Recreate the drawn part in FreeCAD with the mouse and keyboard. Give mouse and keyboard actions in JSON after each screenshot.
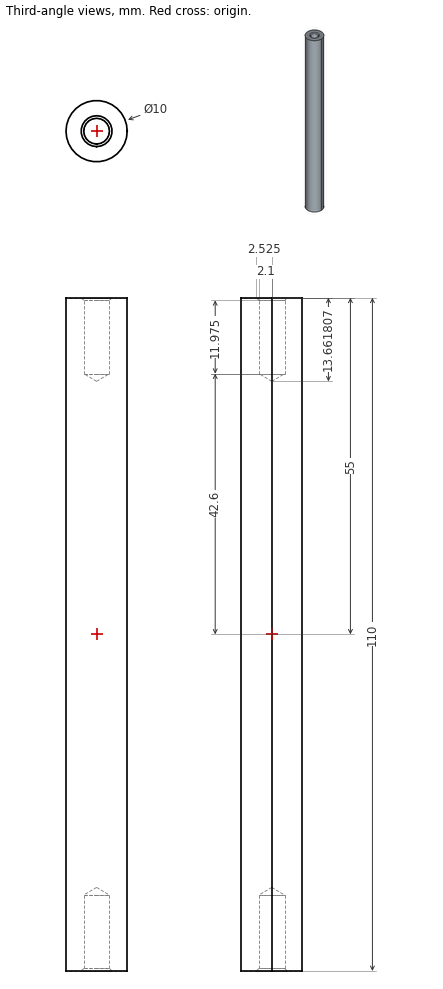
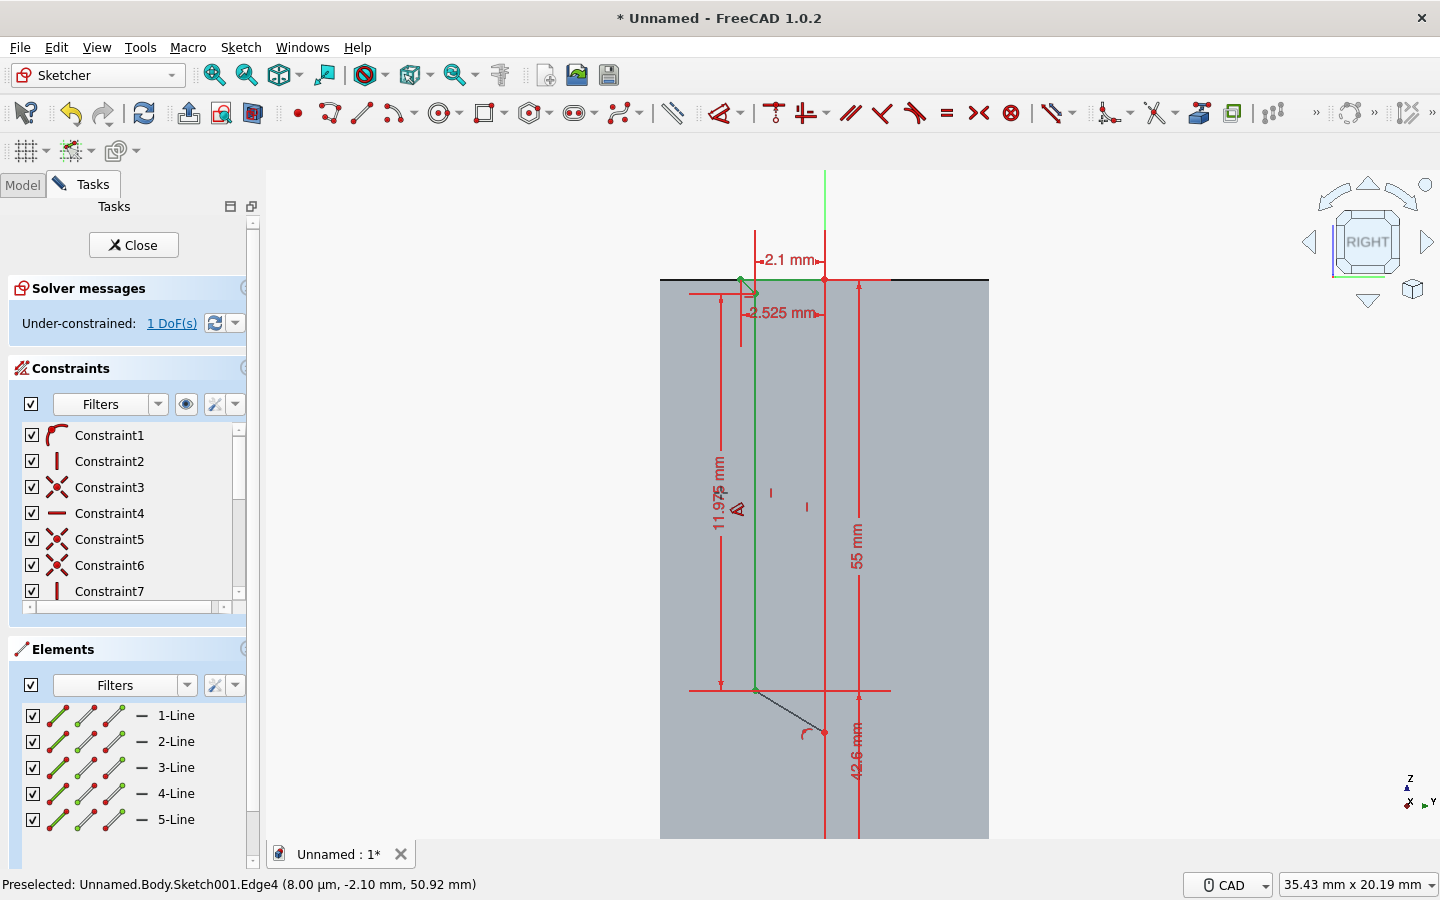
{"action": "left_click", "coordinate": [825, 597]}
{"action": "left_click", "coordinate": [859, 506]}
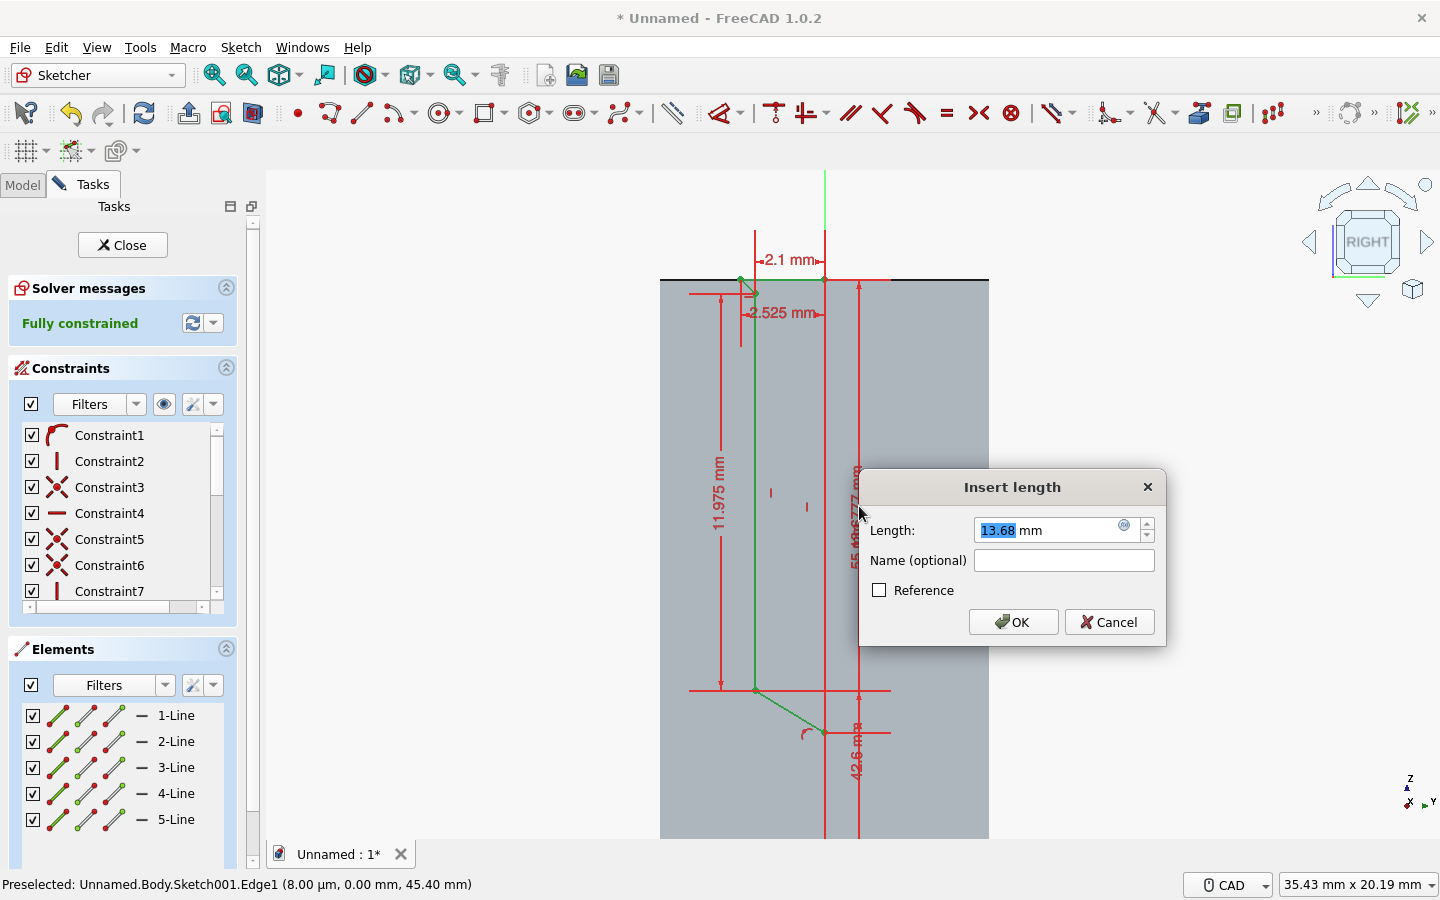
{"action": "type", "text": "13.661807"}
{"action": "key", "text": "Return"}
{"action": "key", "text": "Escape"}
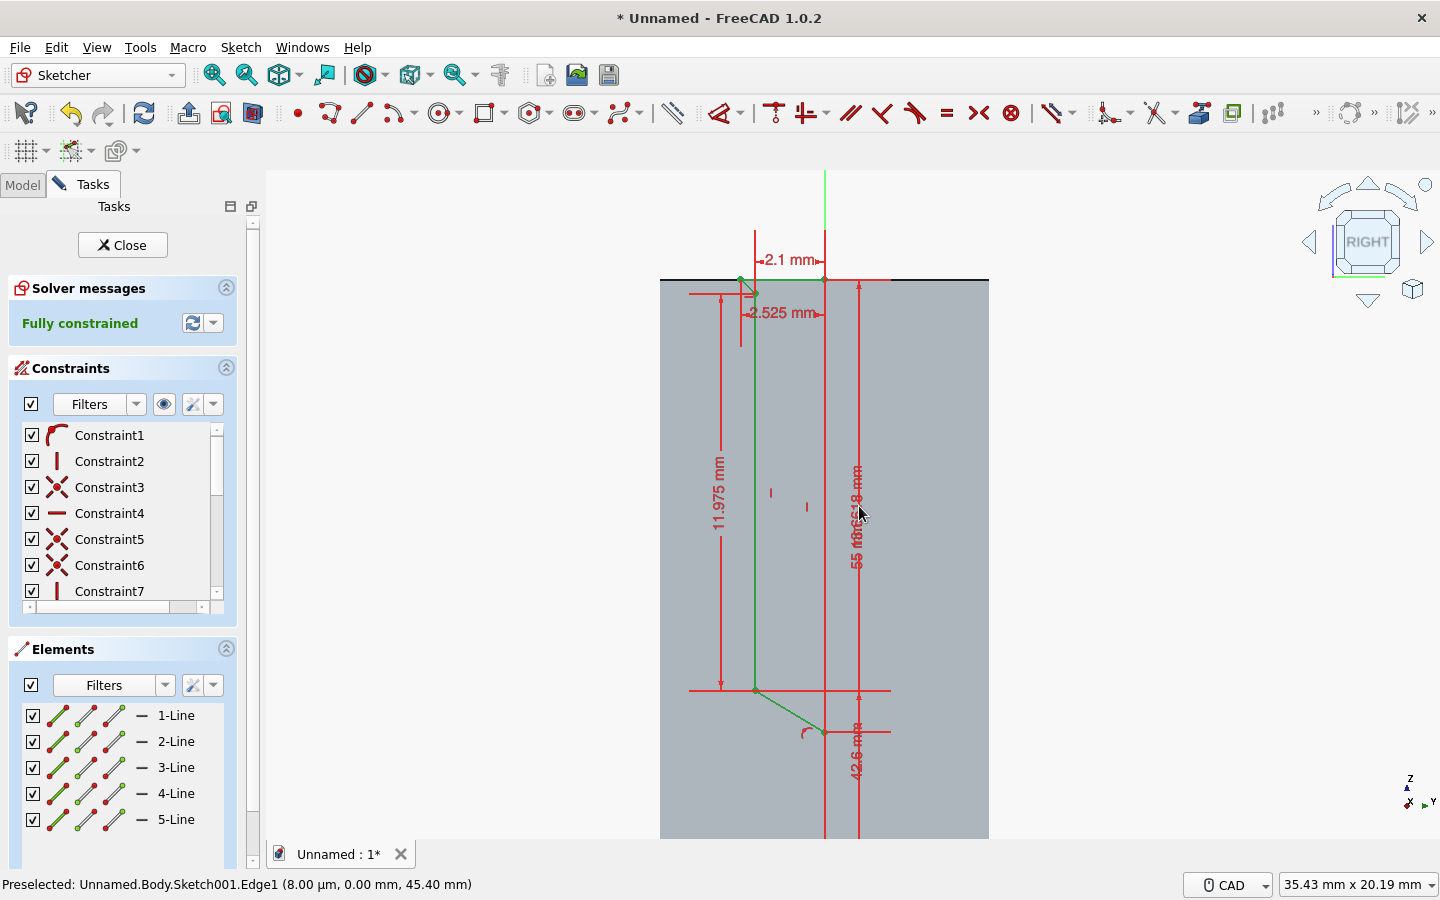
{"action": "left_click", "coordinate": [123, 245]}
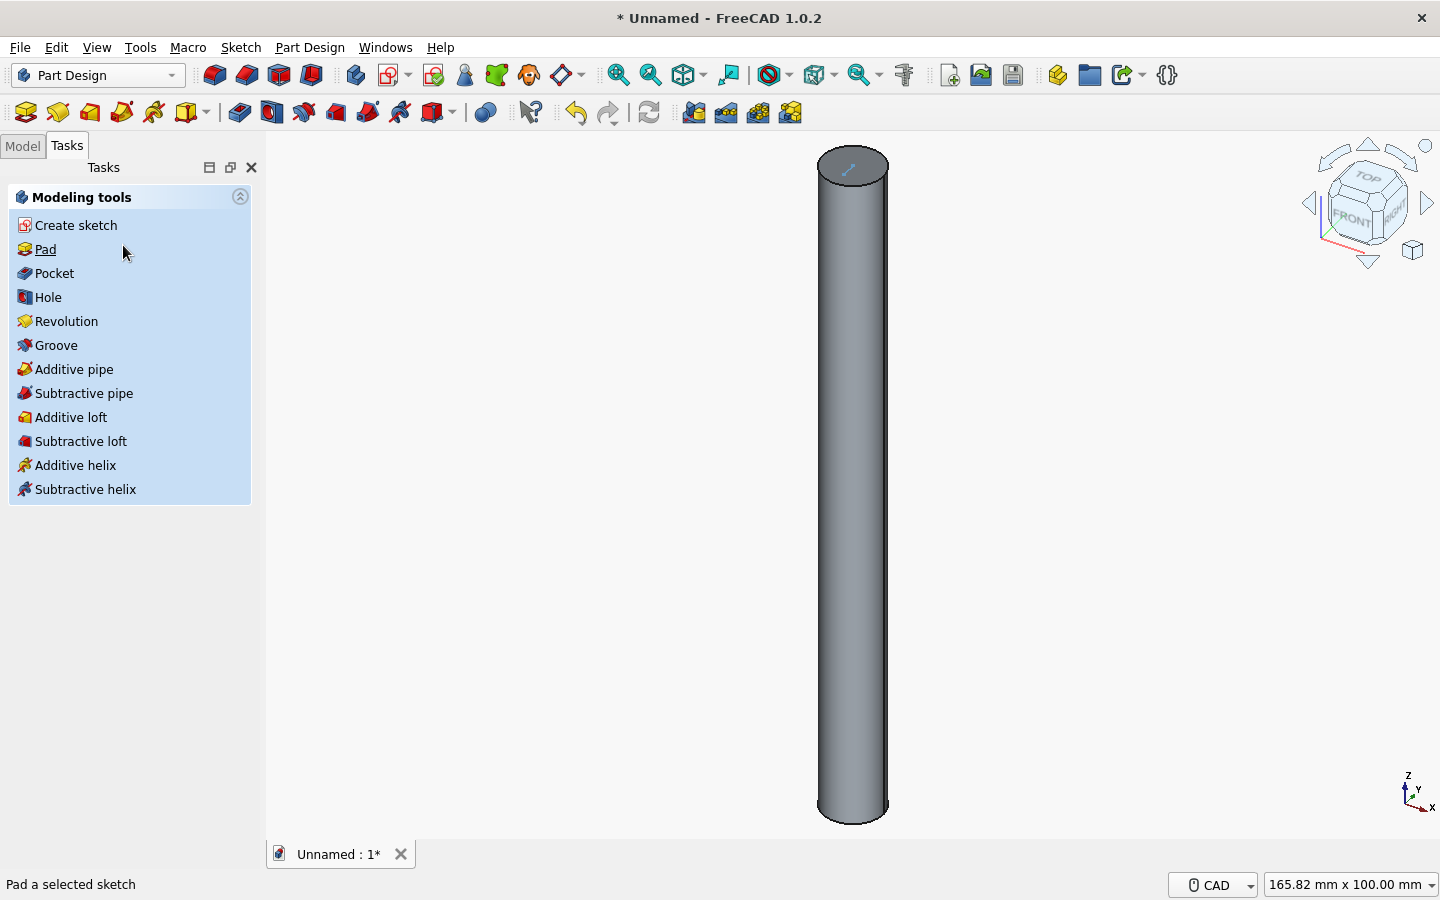
{"action": "left_click", "coordinate": [304, 112]}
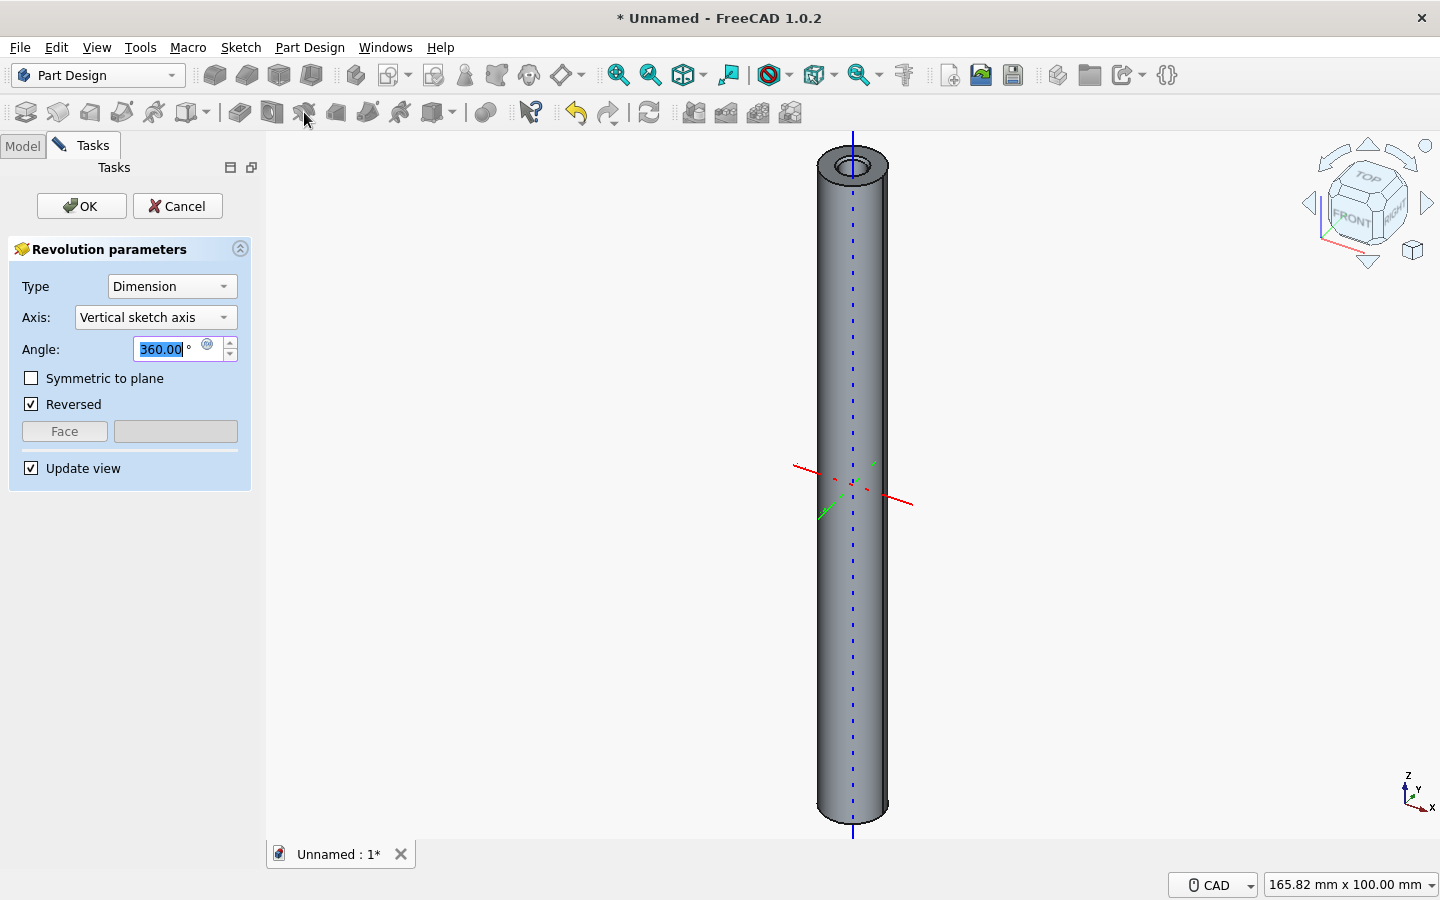
{"action": "left_click", "coordinate": [82, 206]}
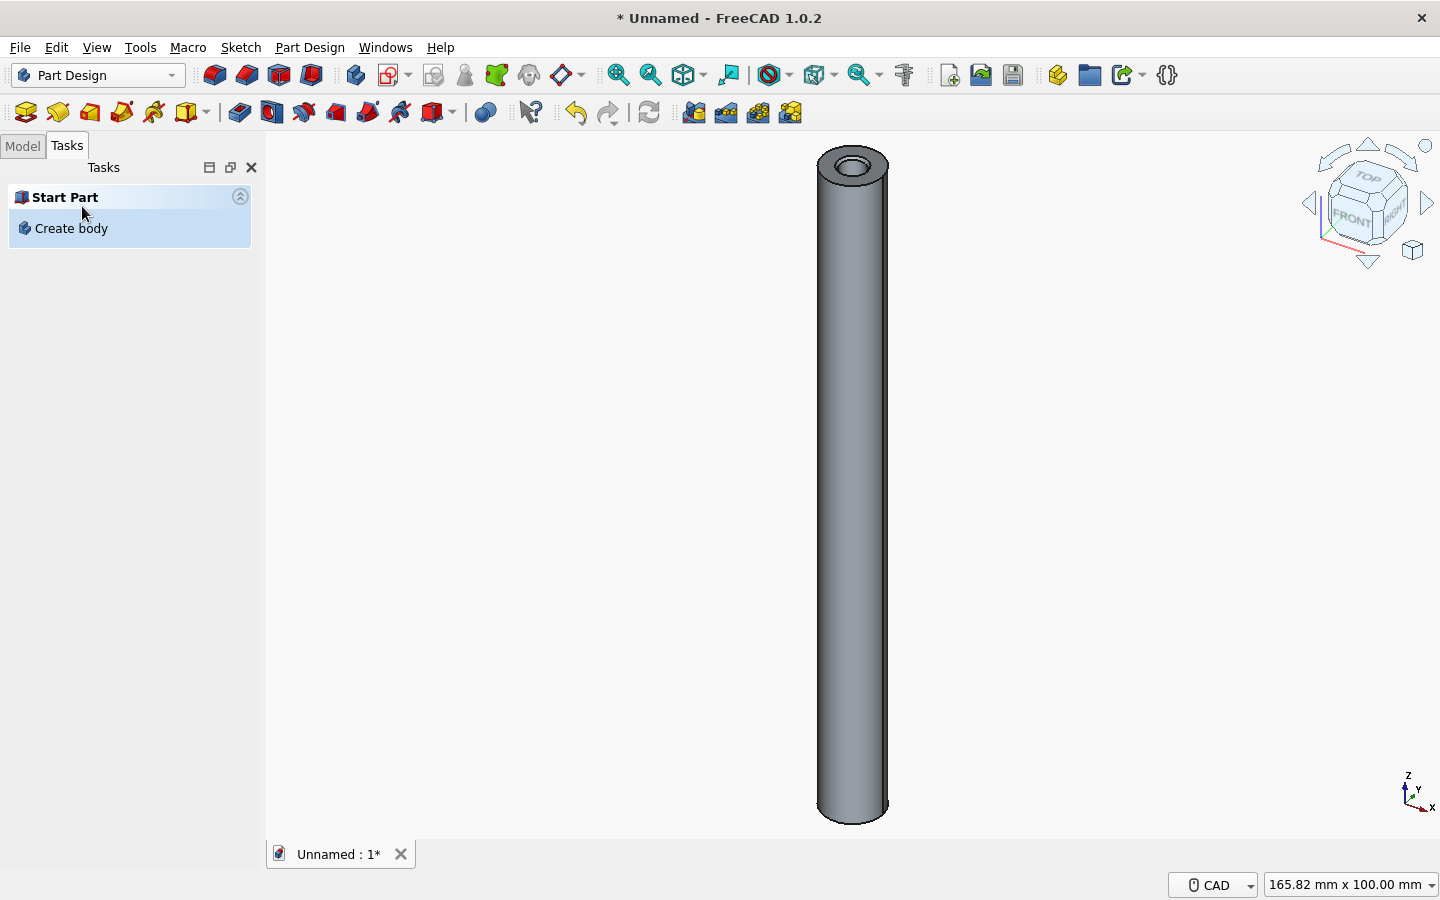
{"action": "left_click", "coordinate": [23, 145]}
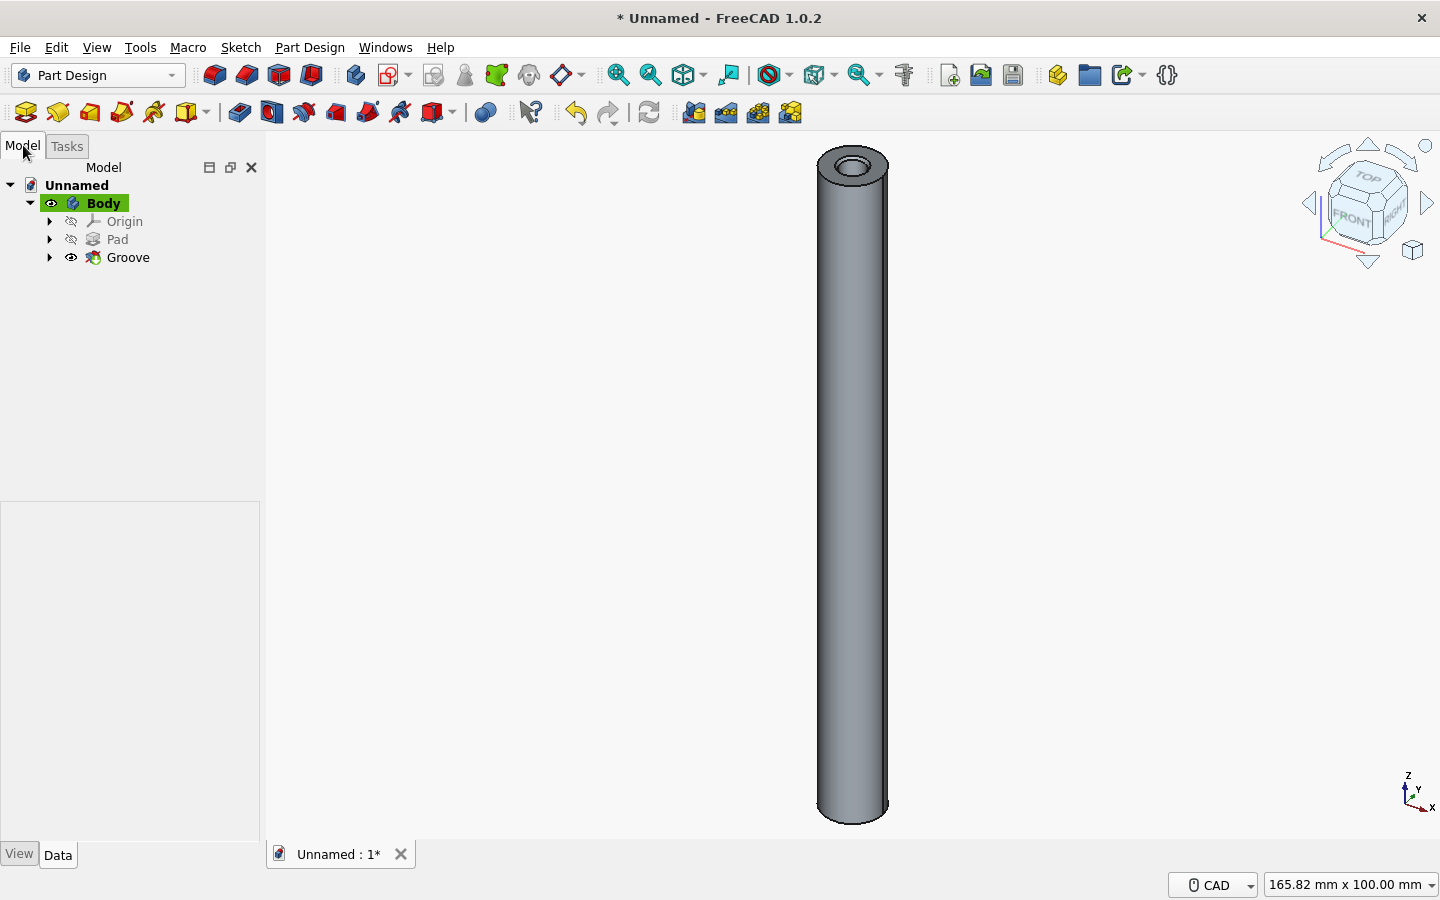
{"action": "left_click", "coordinate": [116, 257]}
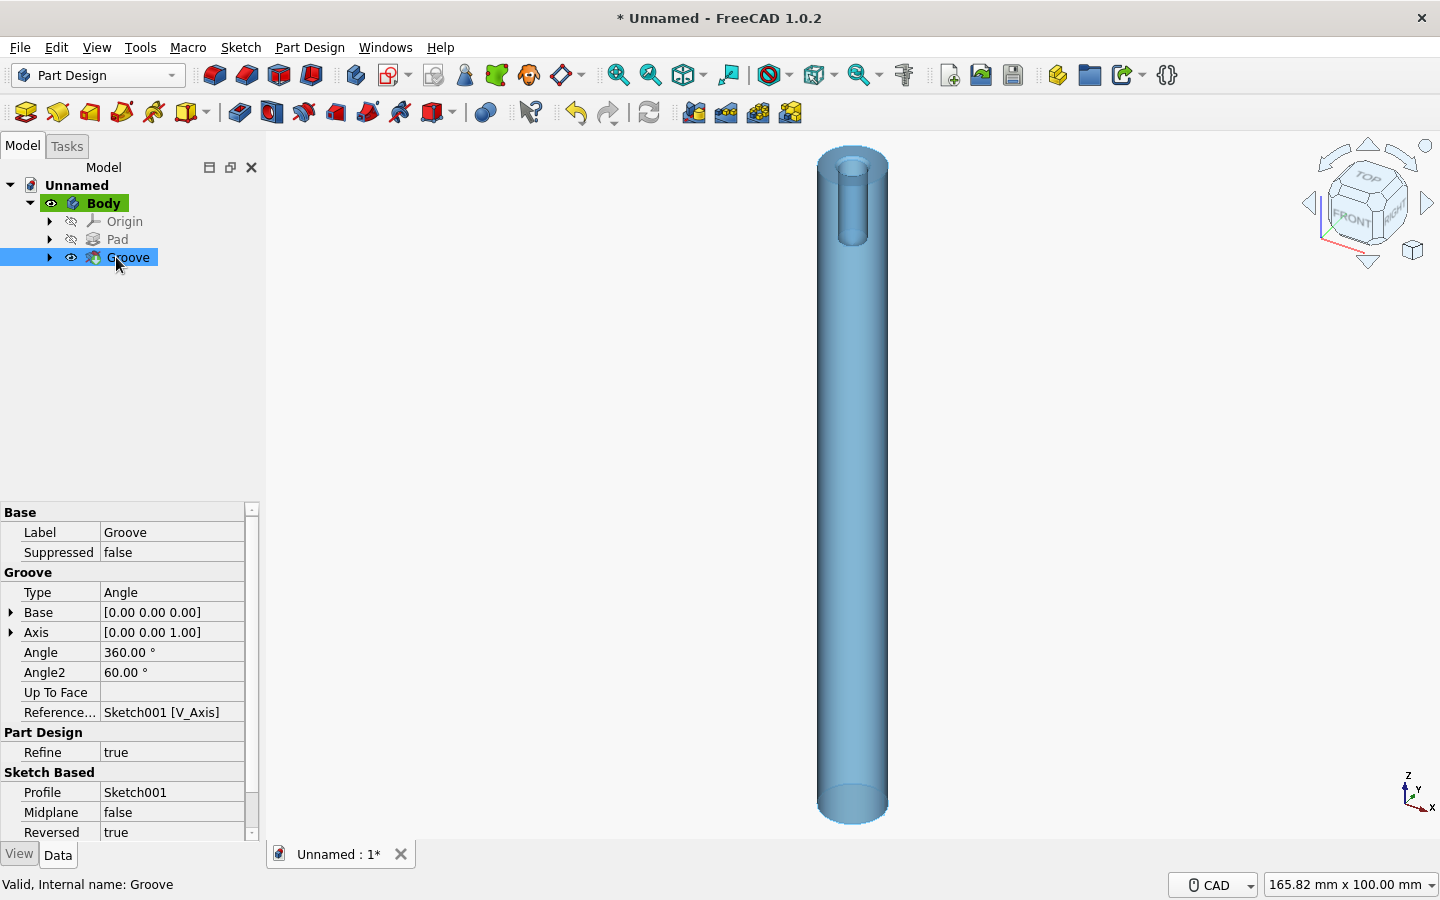
{"action": "left_click", "coordinate": [694, 112]}